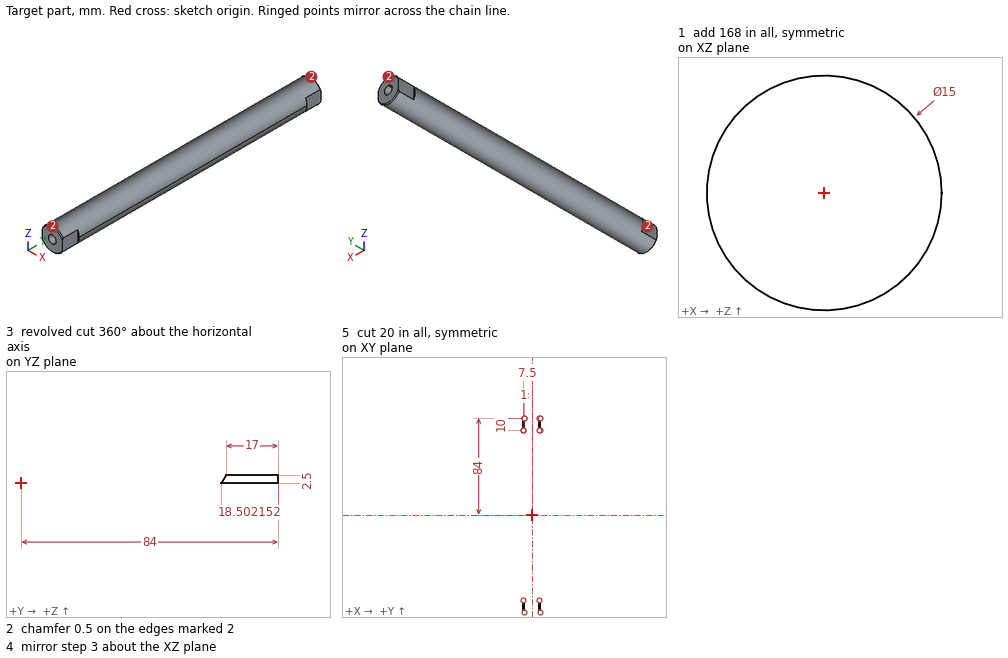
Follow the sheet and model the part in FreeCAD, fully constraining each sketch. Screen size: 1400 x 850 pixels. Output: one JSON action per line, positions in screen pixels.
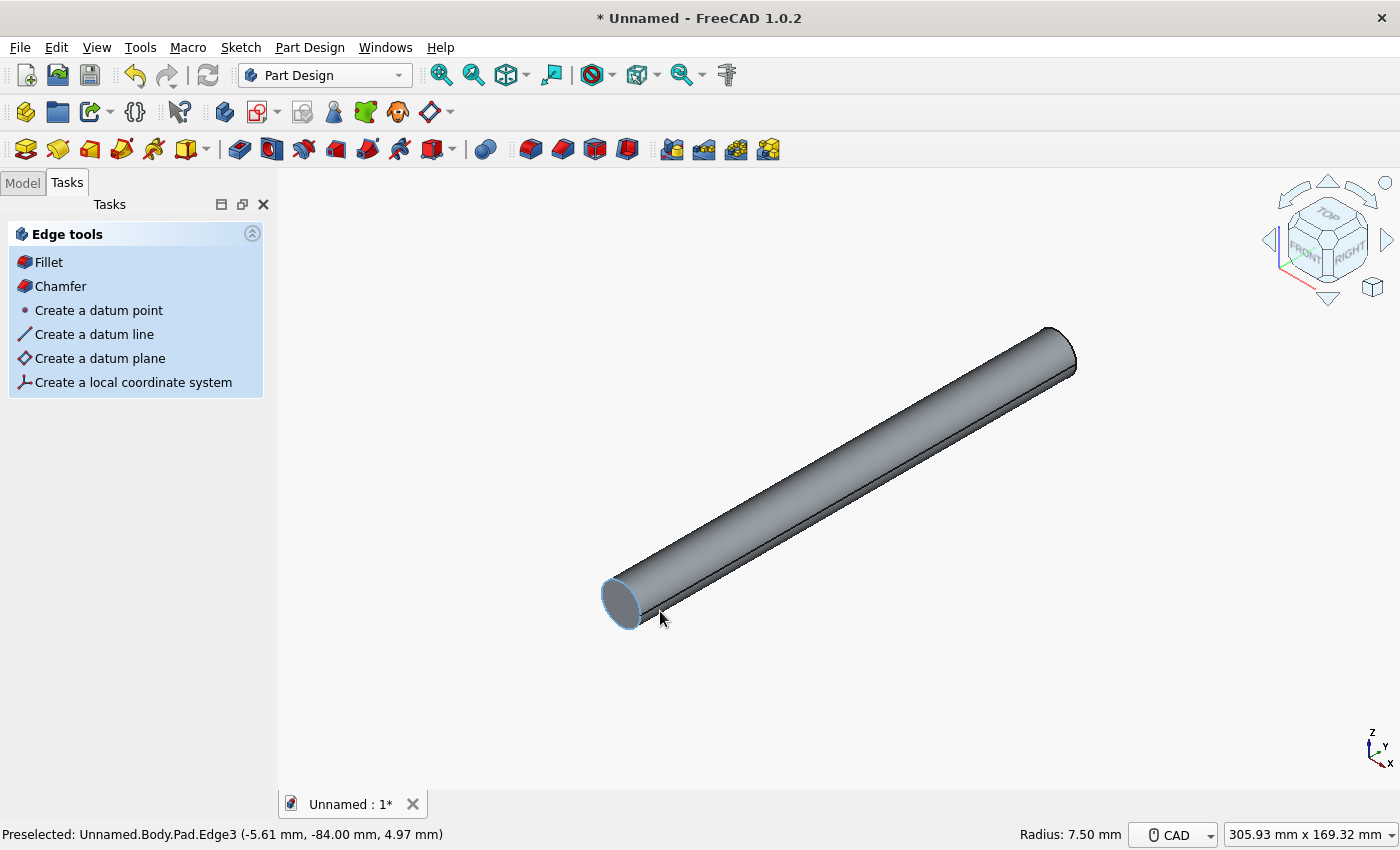
{"action": "key", "text": "2"}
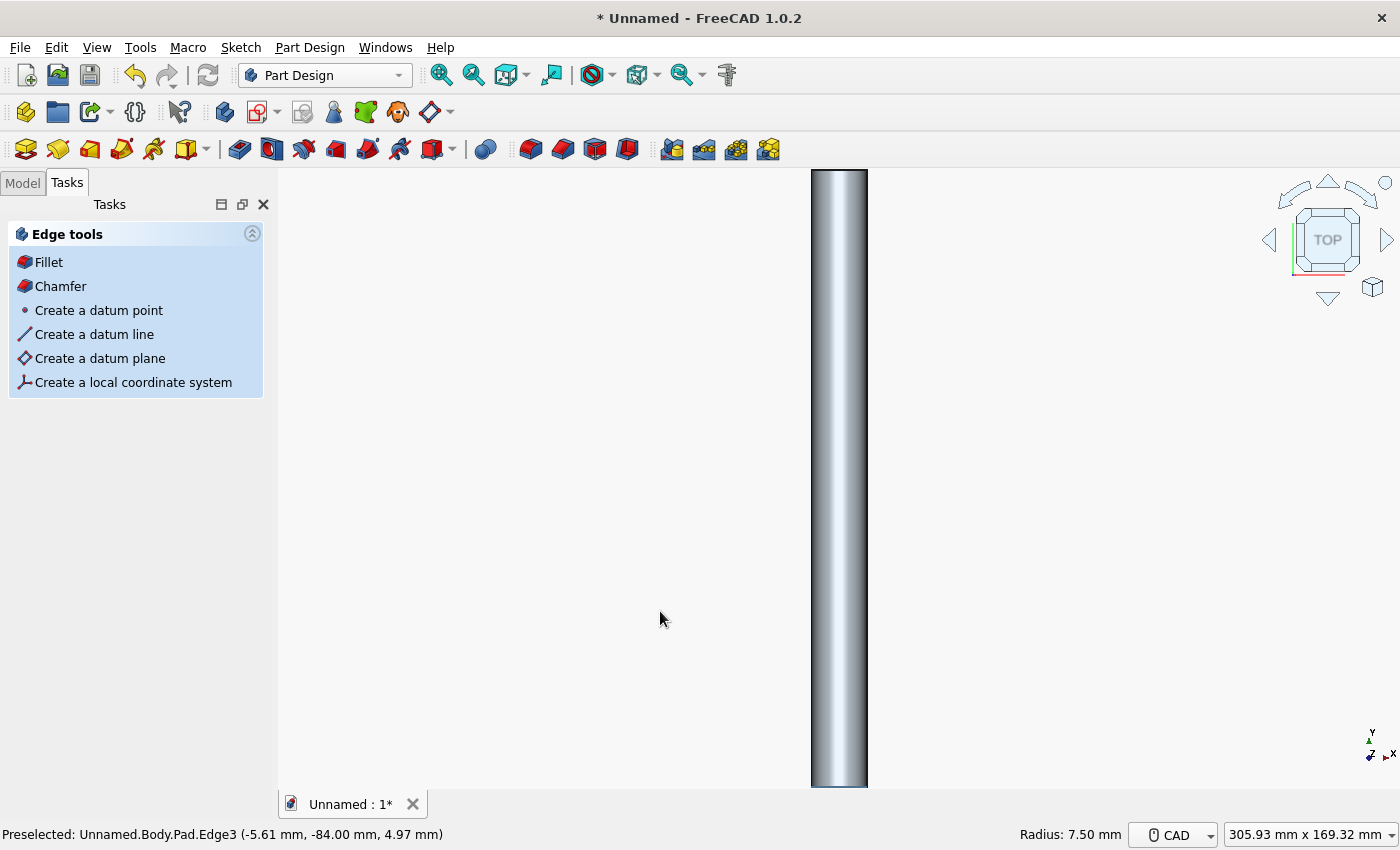
{"action": "key", "text": "1"}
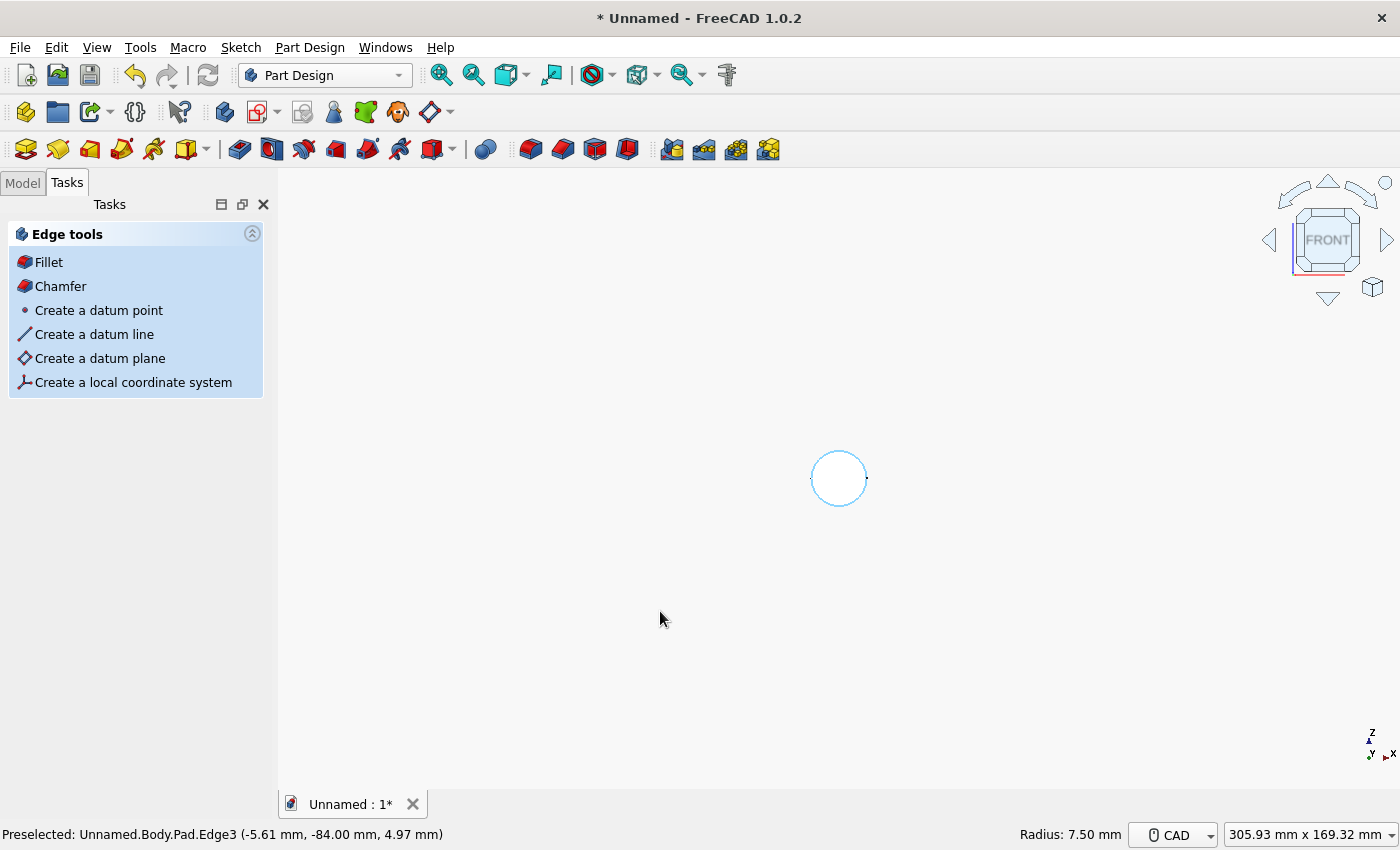
{"action": "left_click", "coordinate": [442, 76]}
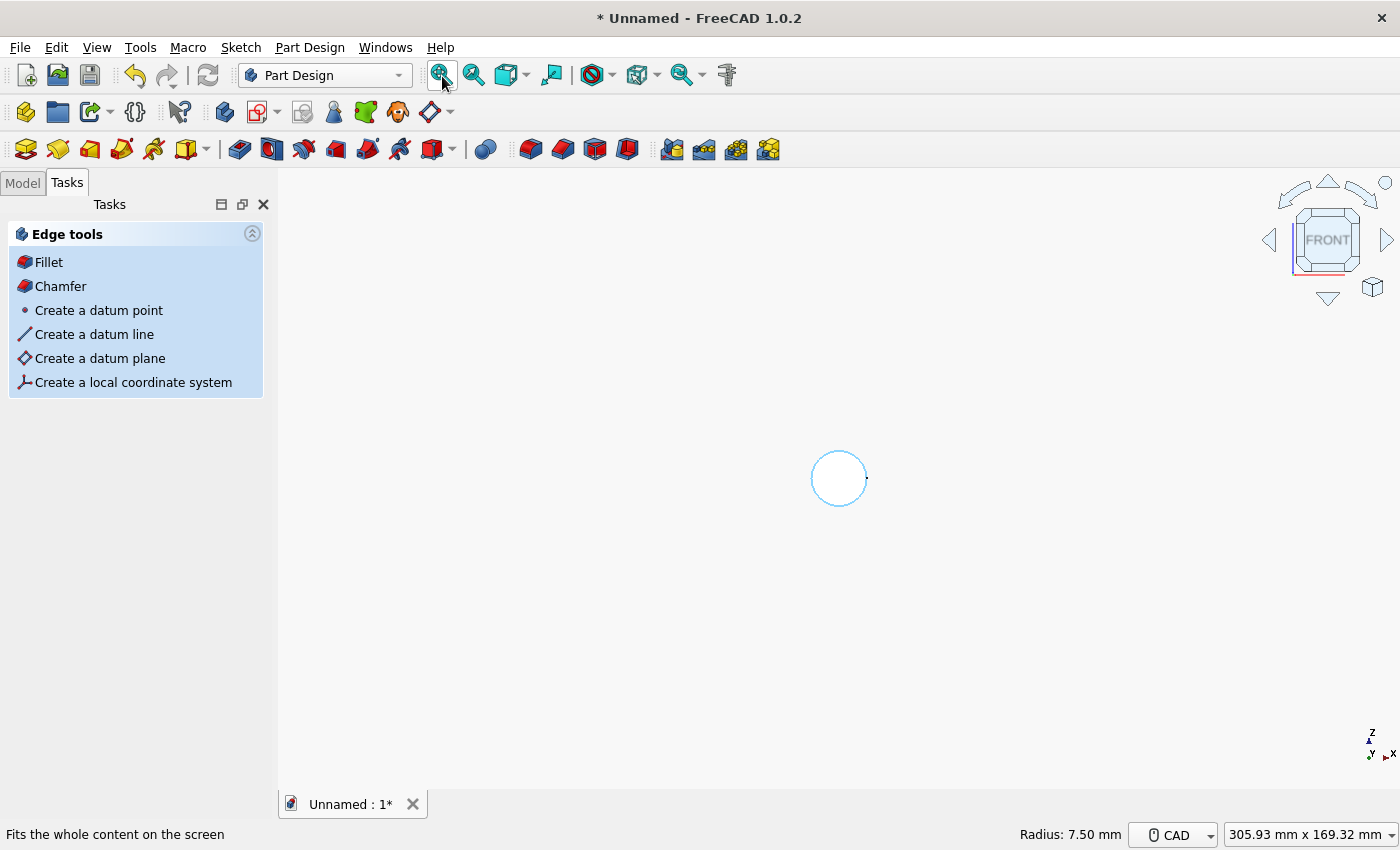
{"action": "key", "text": "3"}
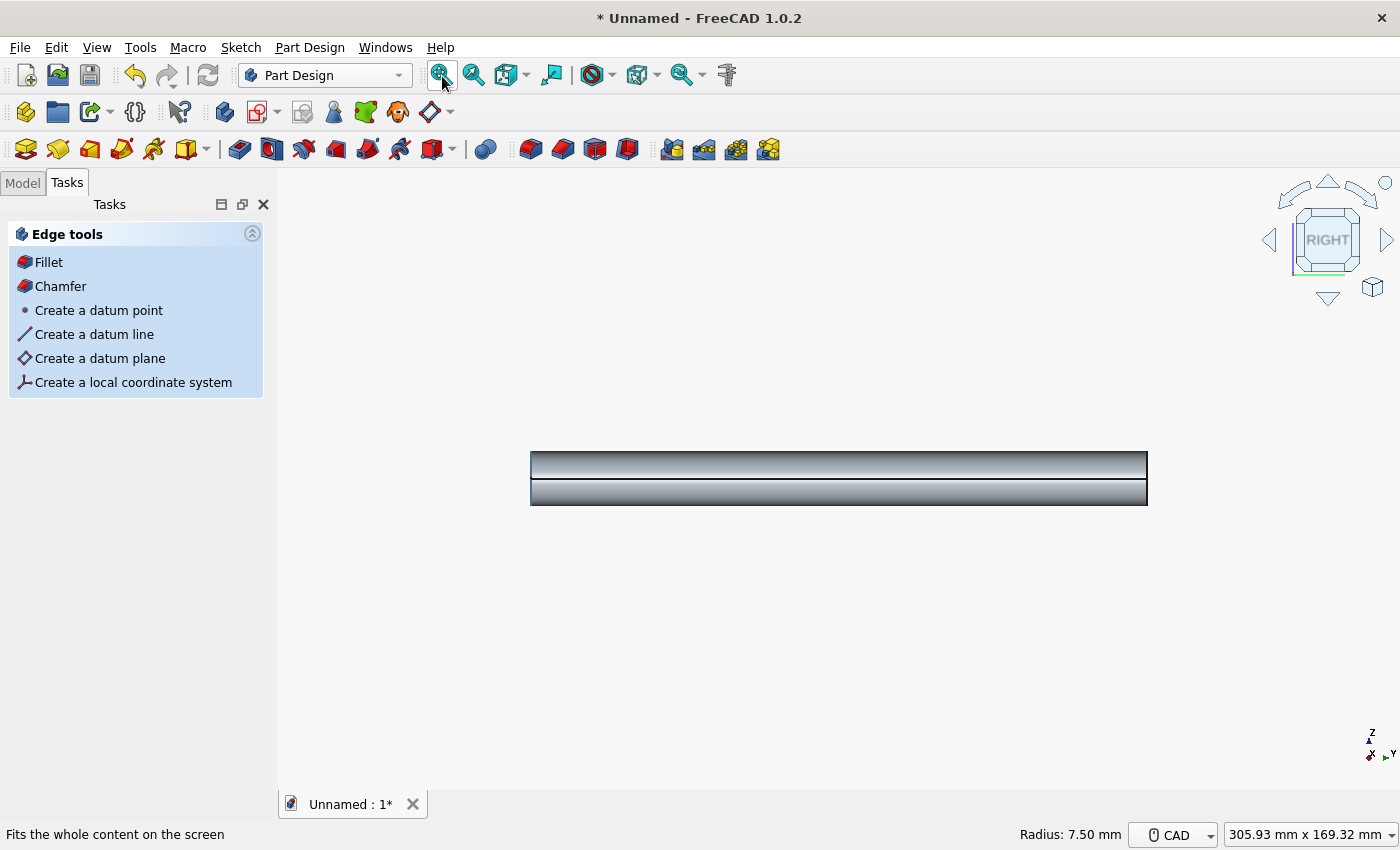
{"action": "left_click", "coordinate": [1147, 461], "text": "ctrl"}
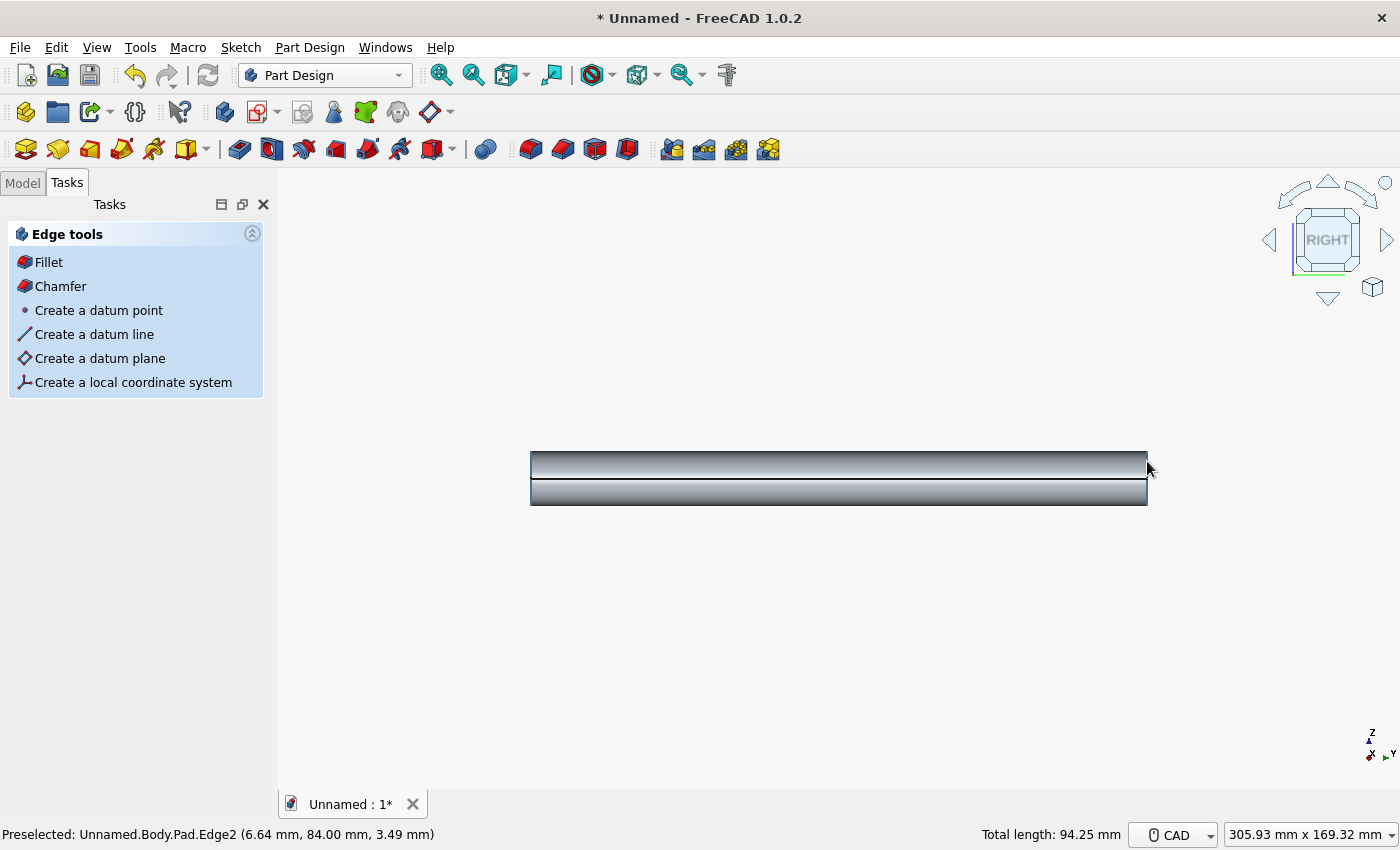
{"action": "left_click", "coordinate": [564, 150]}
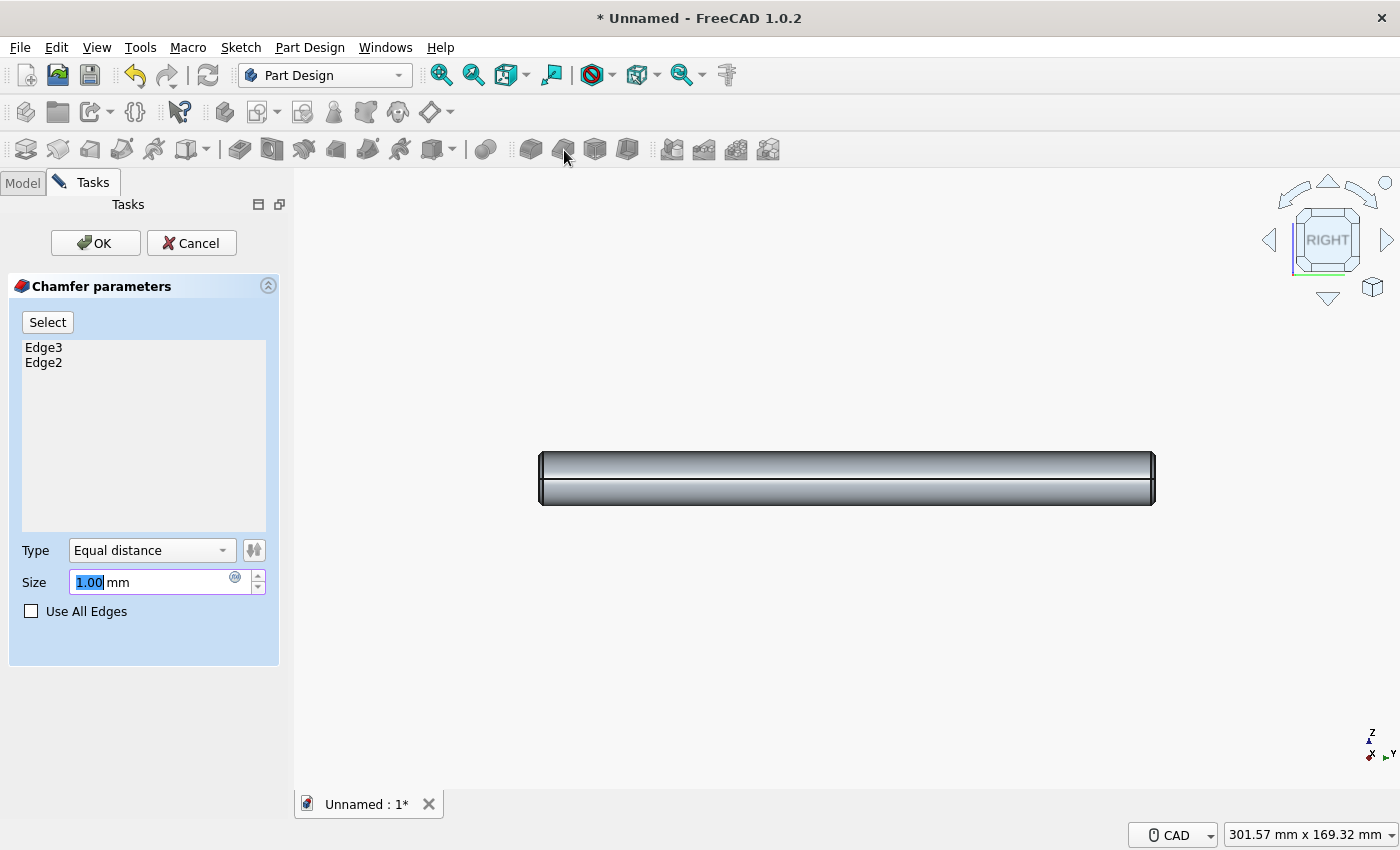
{"action": "type", "text": "0.5"}
{"action": "key", "text": "Tab"}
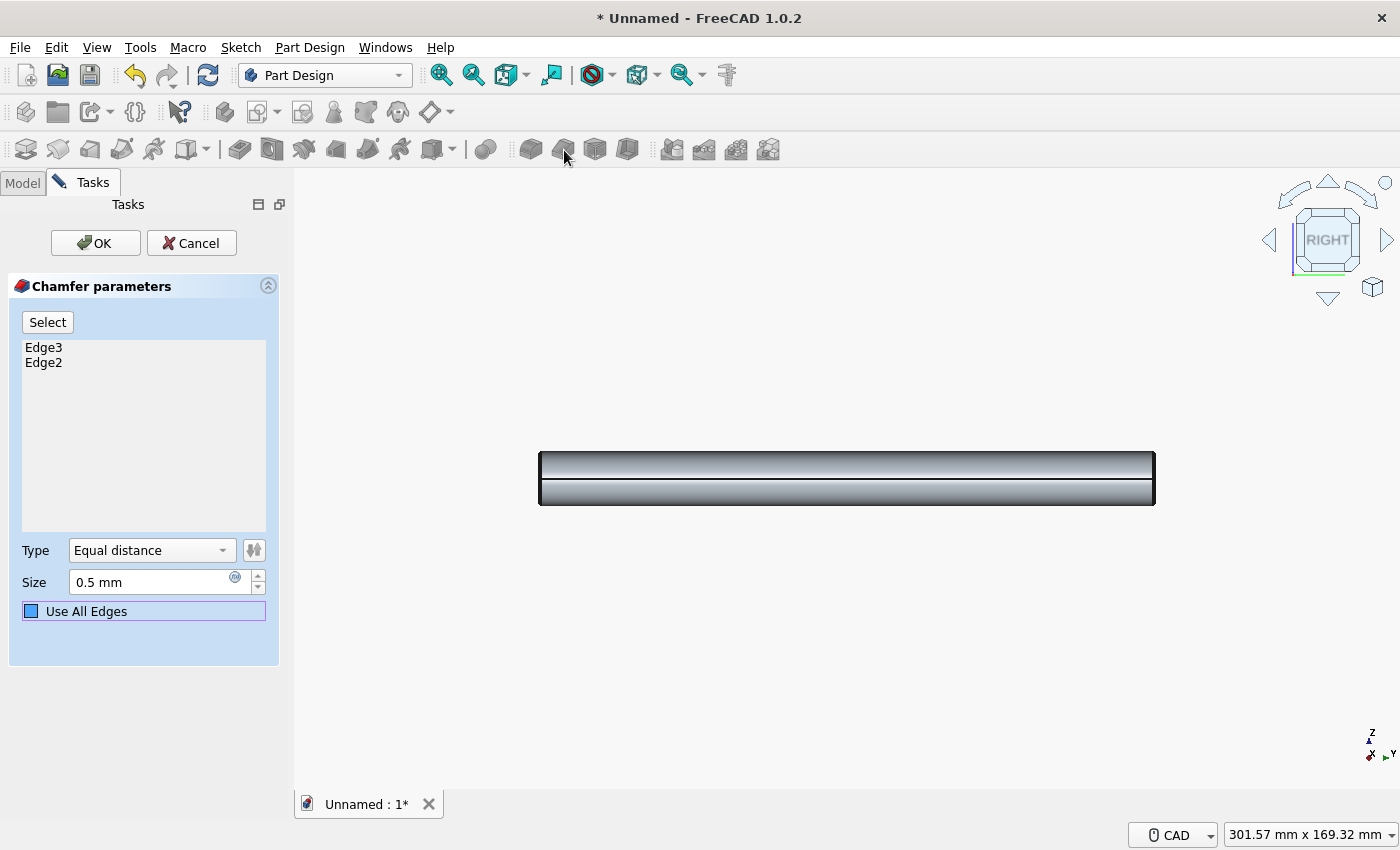
{"action": "left_click", "coordinate": [96, 243]}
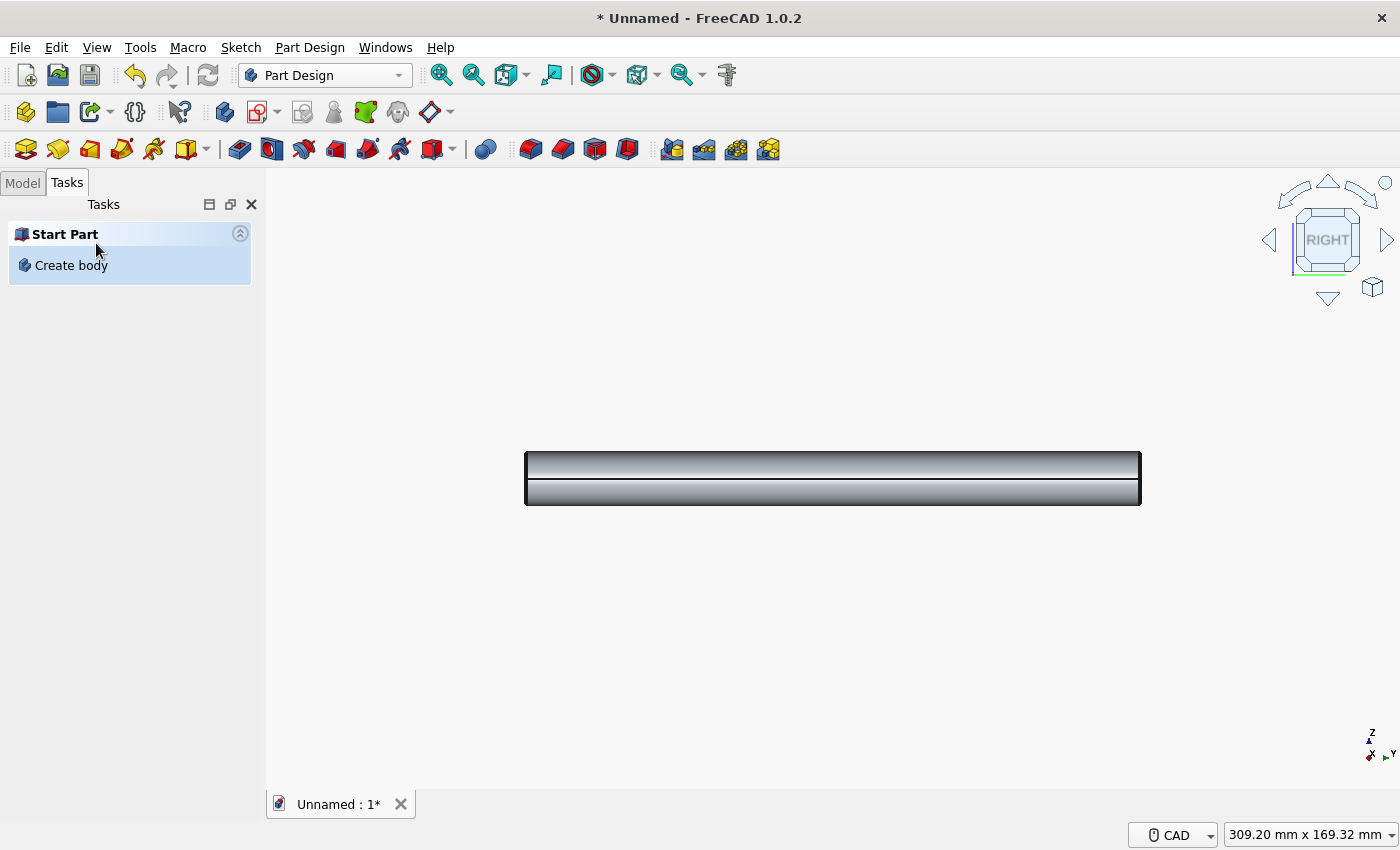
{"action": "left_click", "coordinate": [258, 112]}